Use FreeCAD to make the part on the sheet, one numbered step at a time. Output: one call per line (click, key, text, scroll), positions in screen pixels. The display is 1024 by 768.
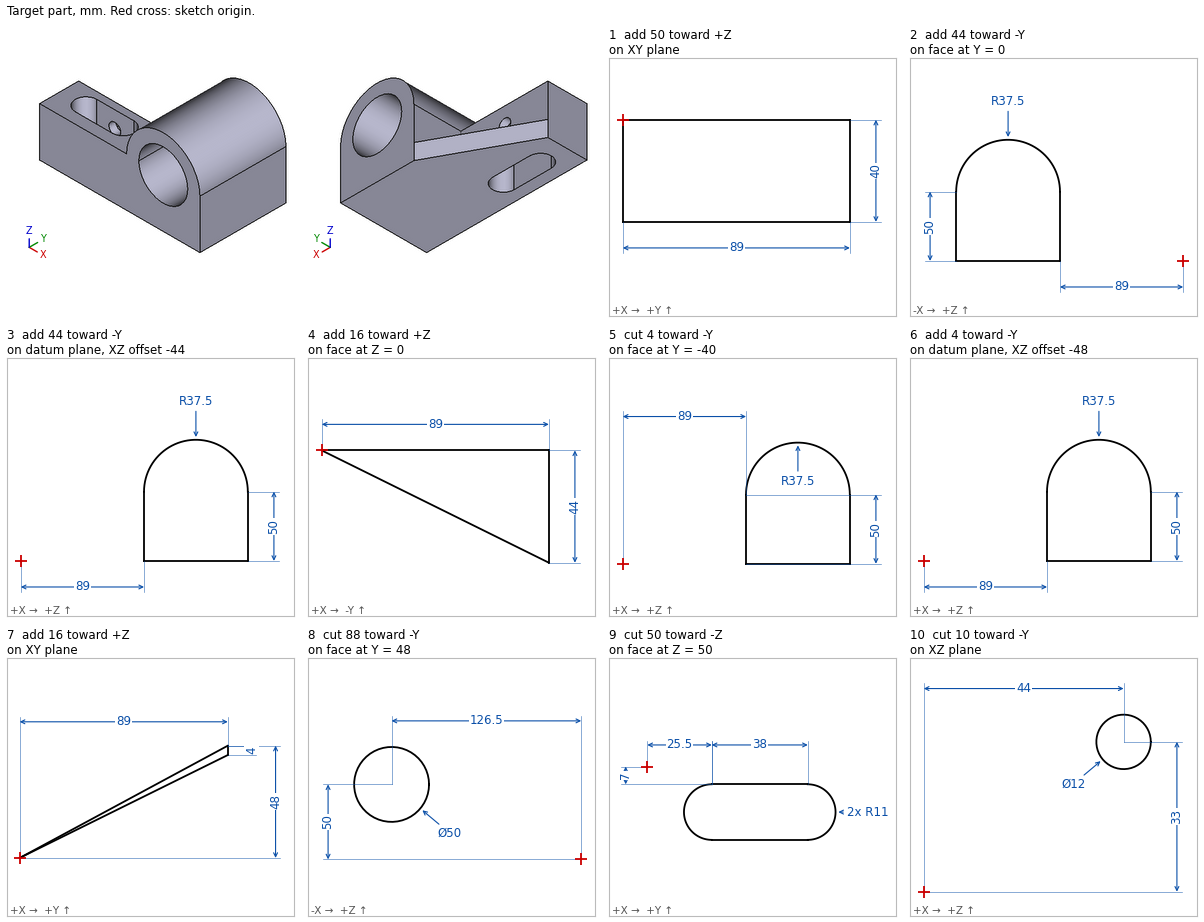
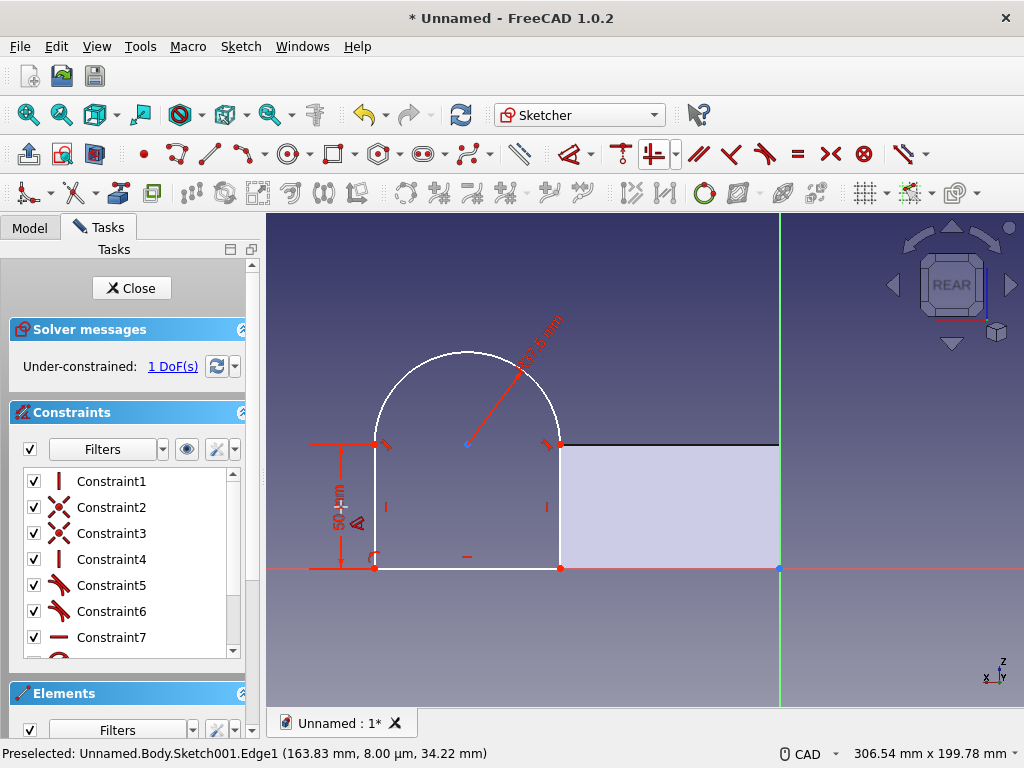
click(560, 569)
click(670, 603)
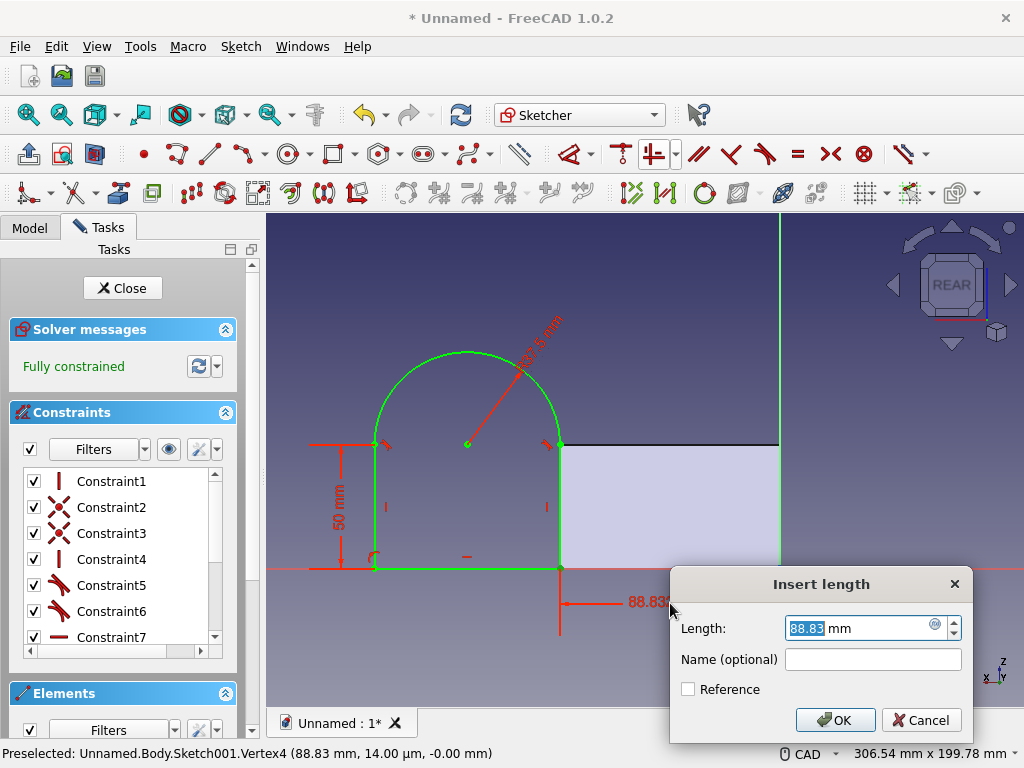
text(89)
key(Return)
key(Escape)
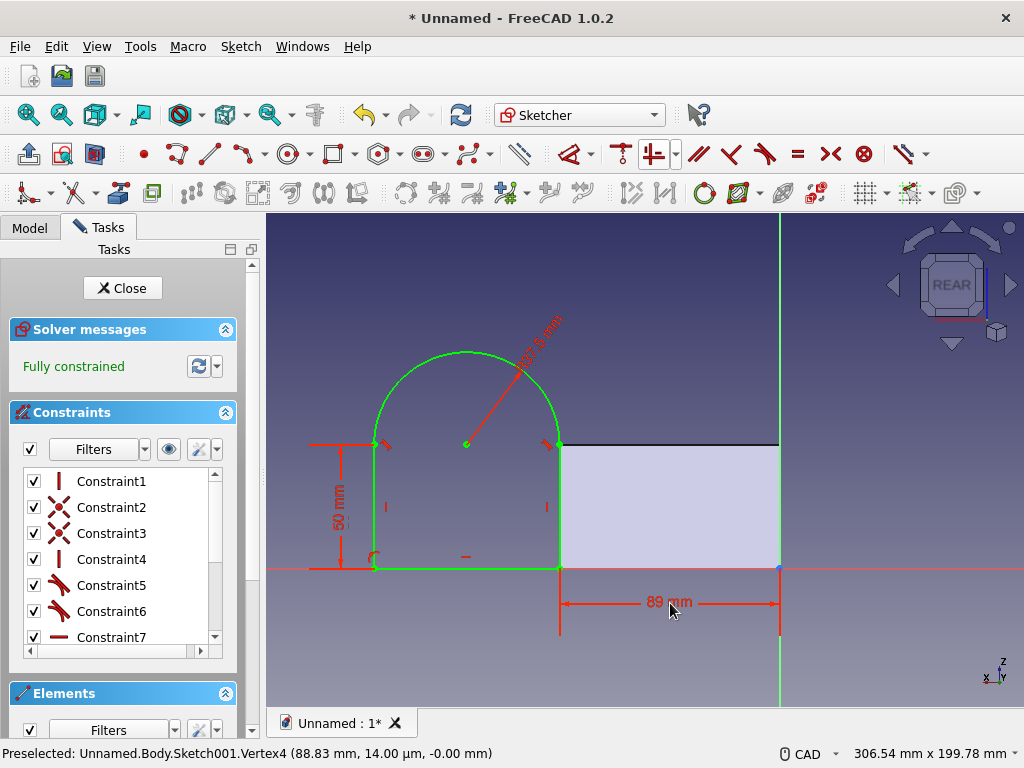
click(123, 288)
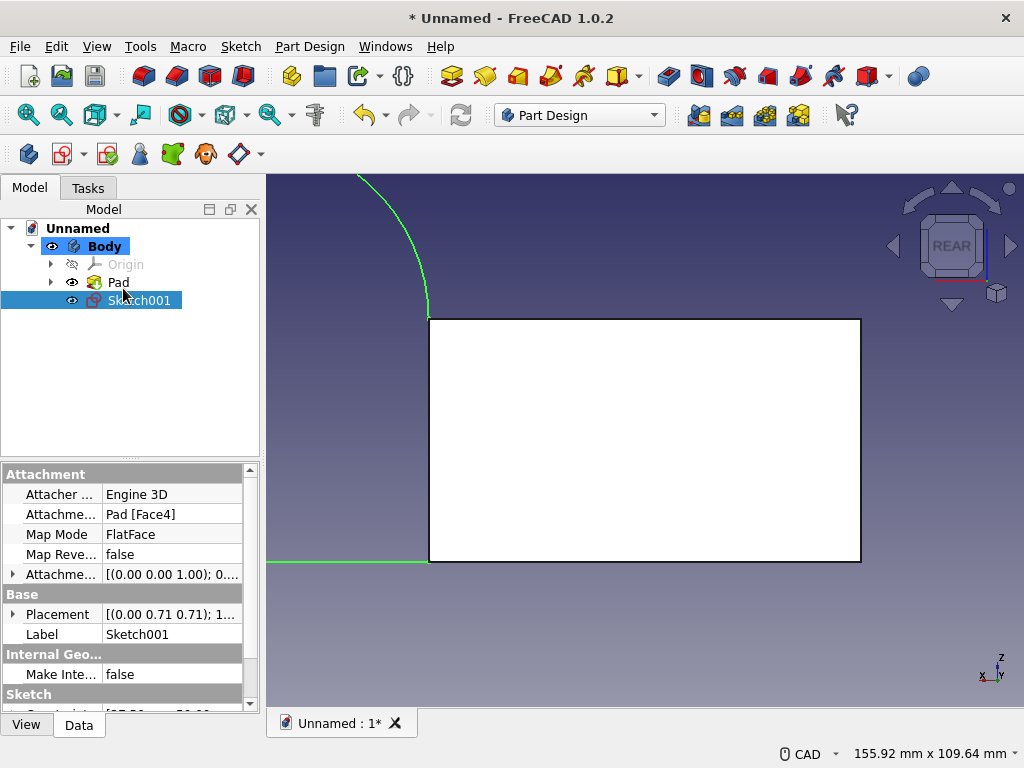
click(452, 76)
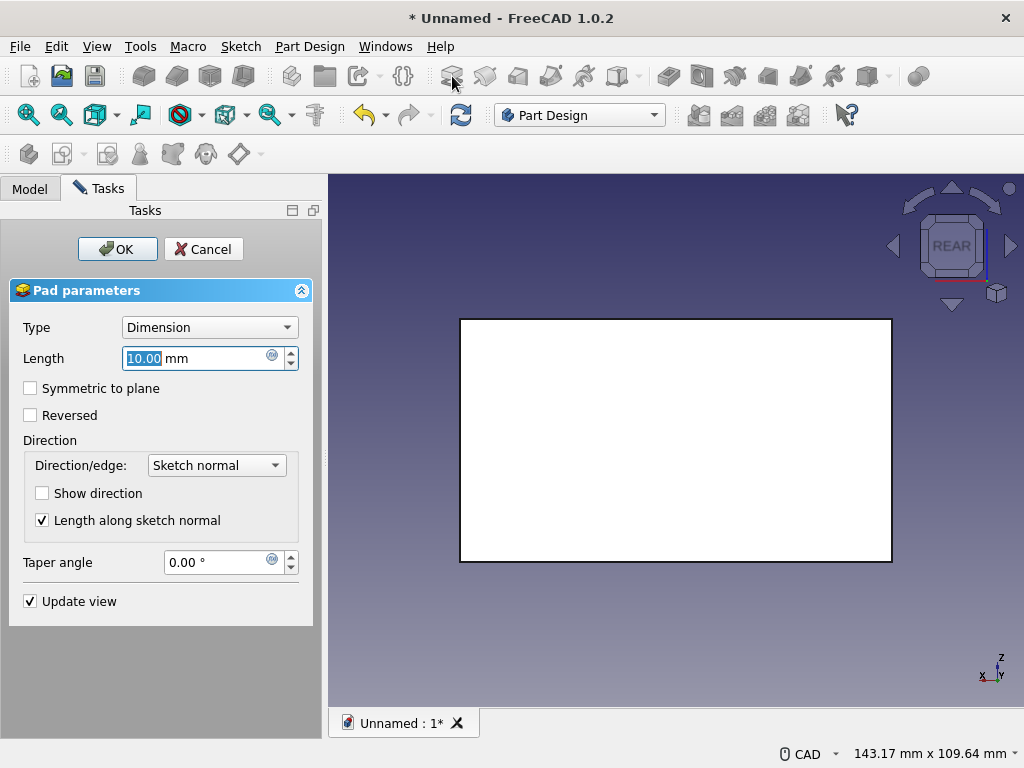
text(44)
key(Tab)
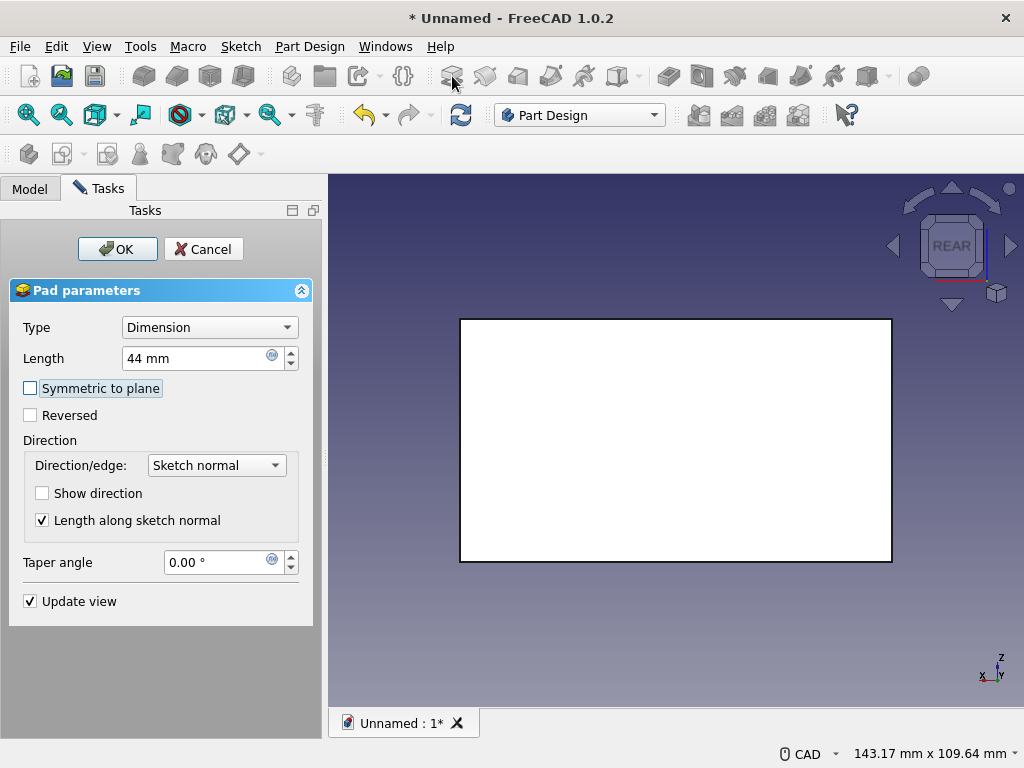
click(31, 415)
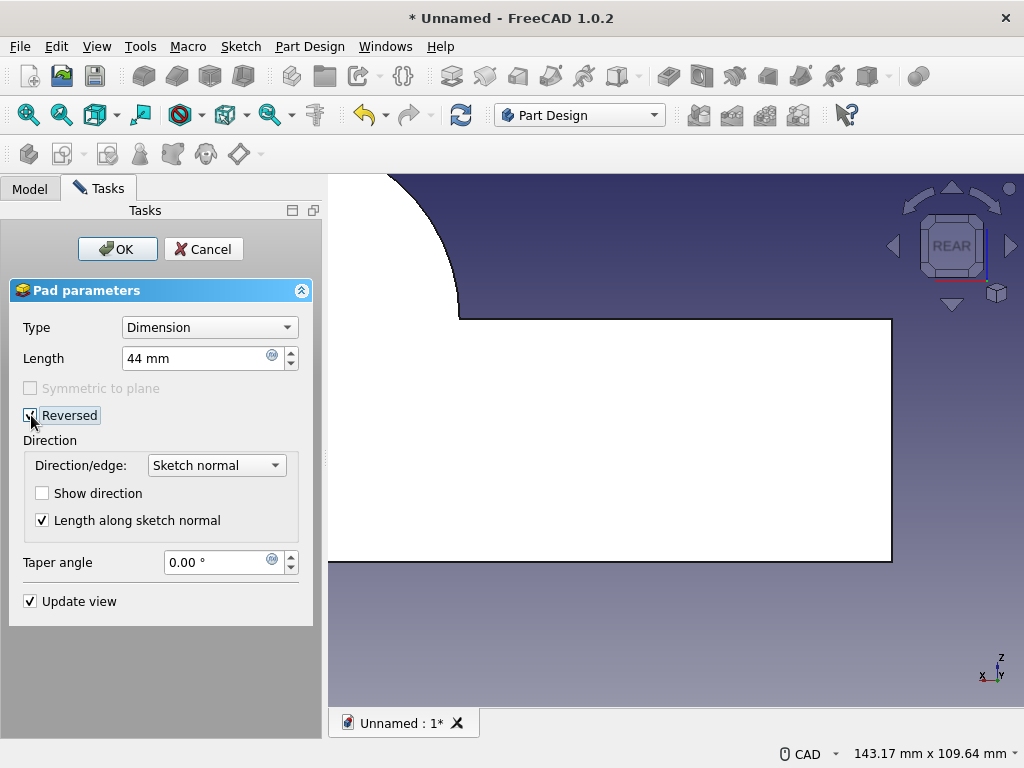
click(118, 249)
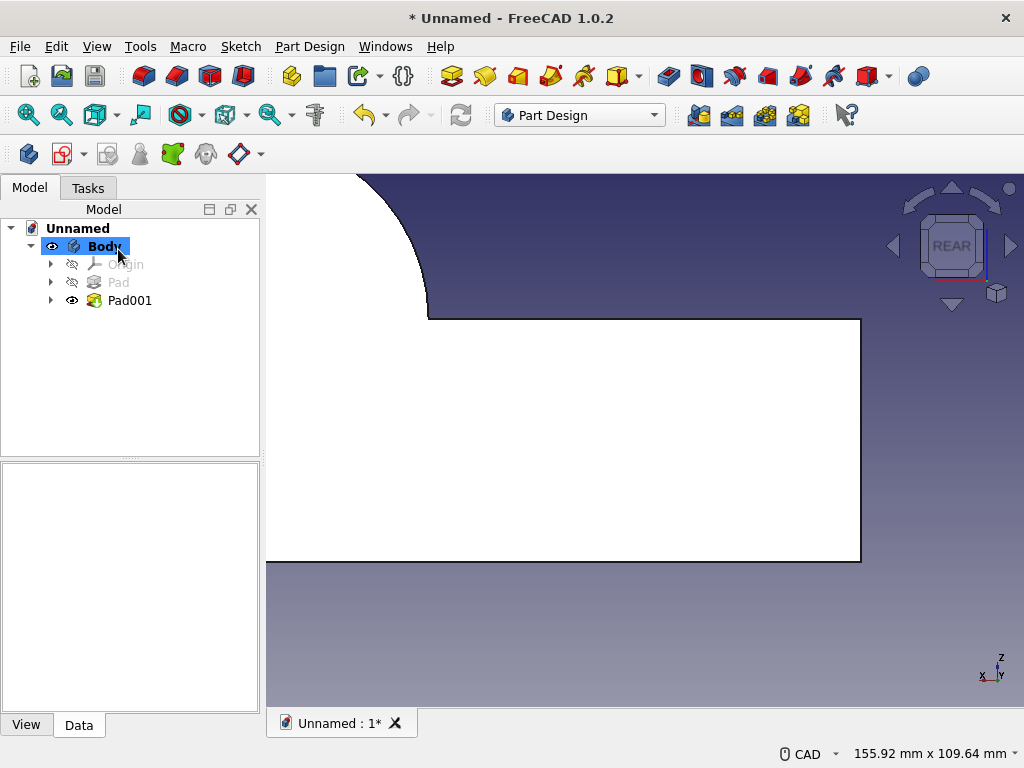
key(v)
key(f)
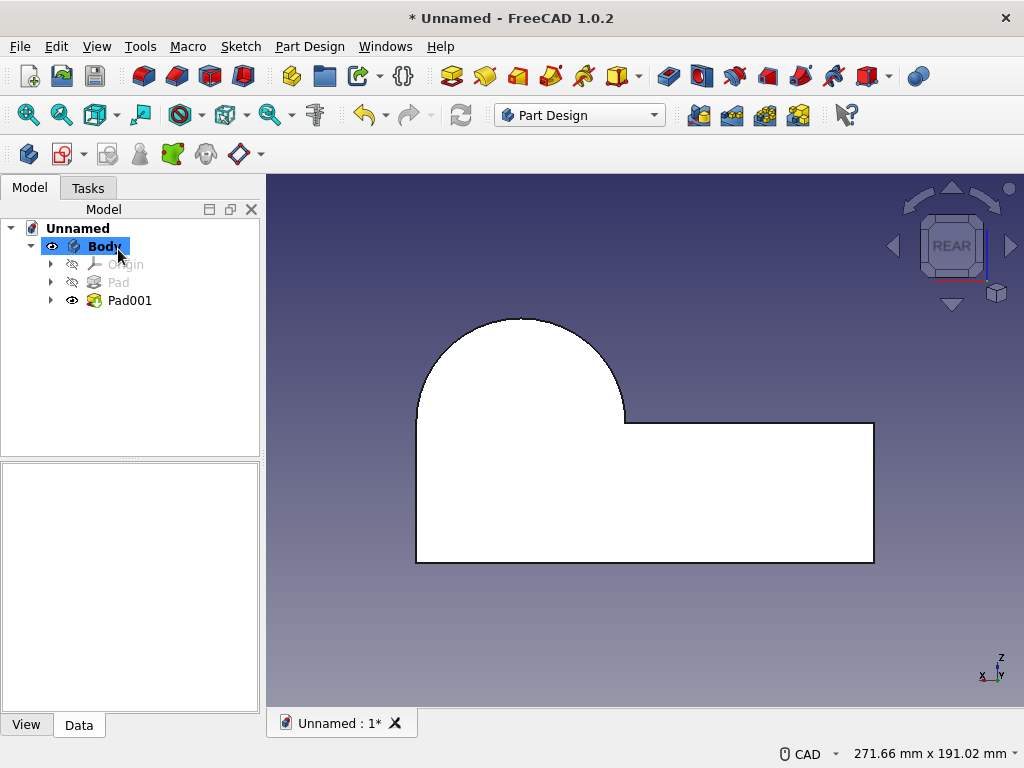
click(51, 264)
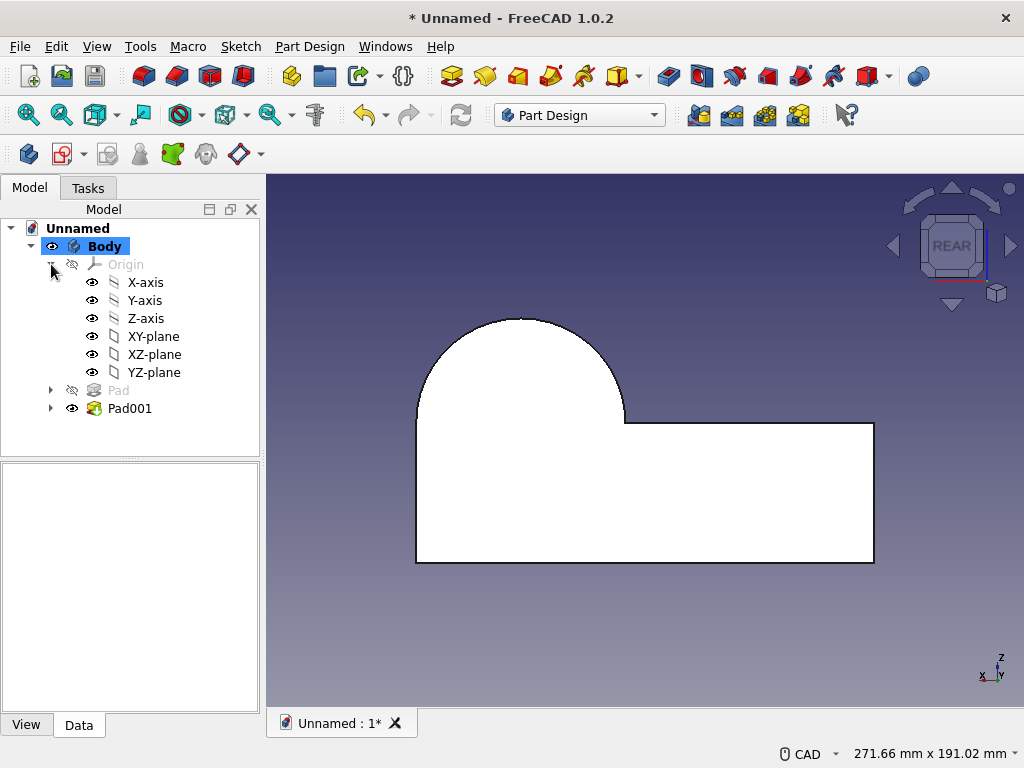
click(137, 354)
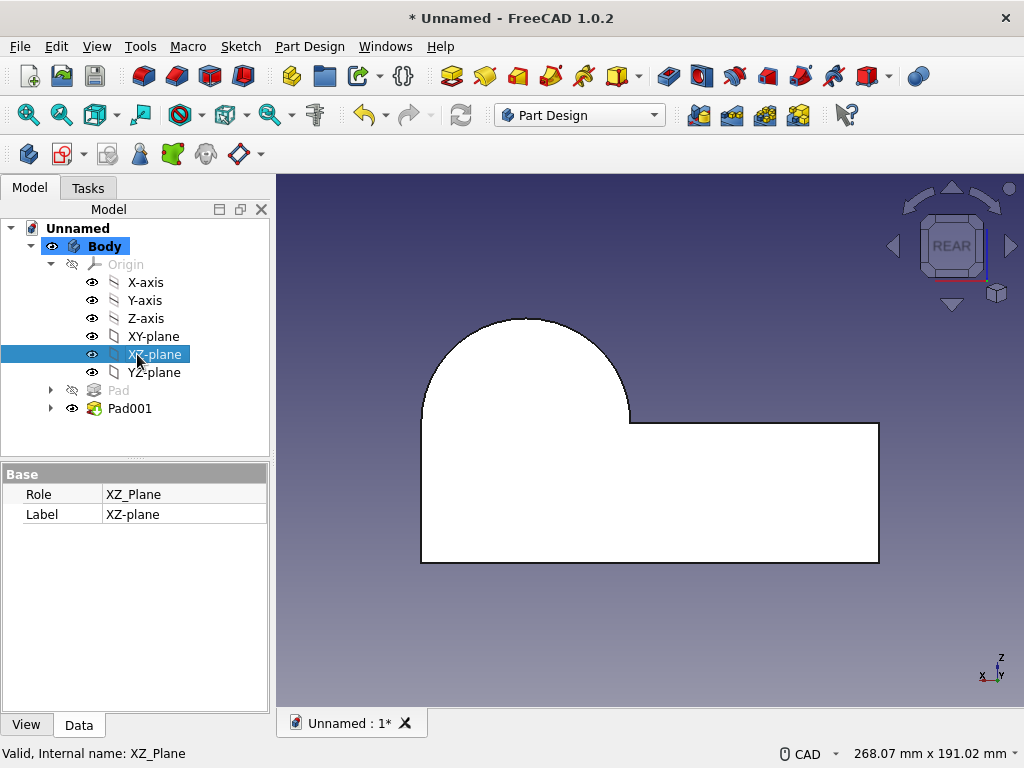
click(238, 154)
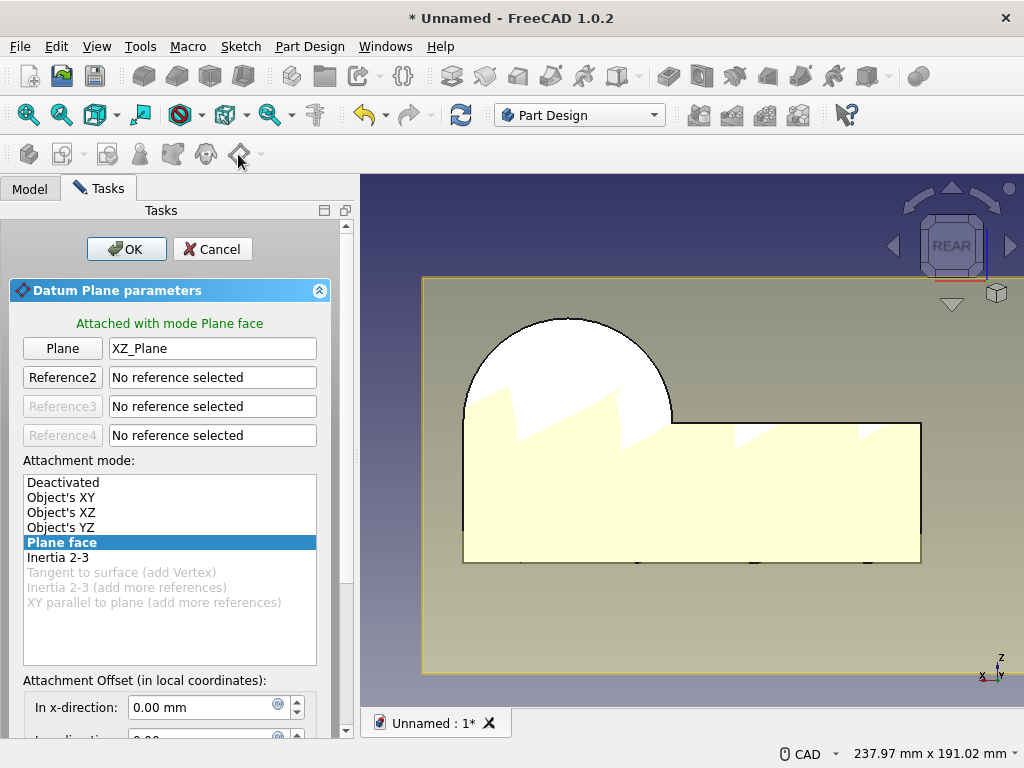
scroll(346, 479, down, 2)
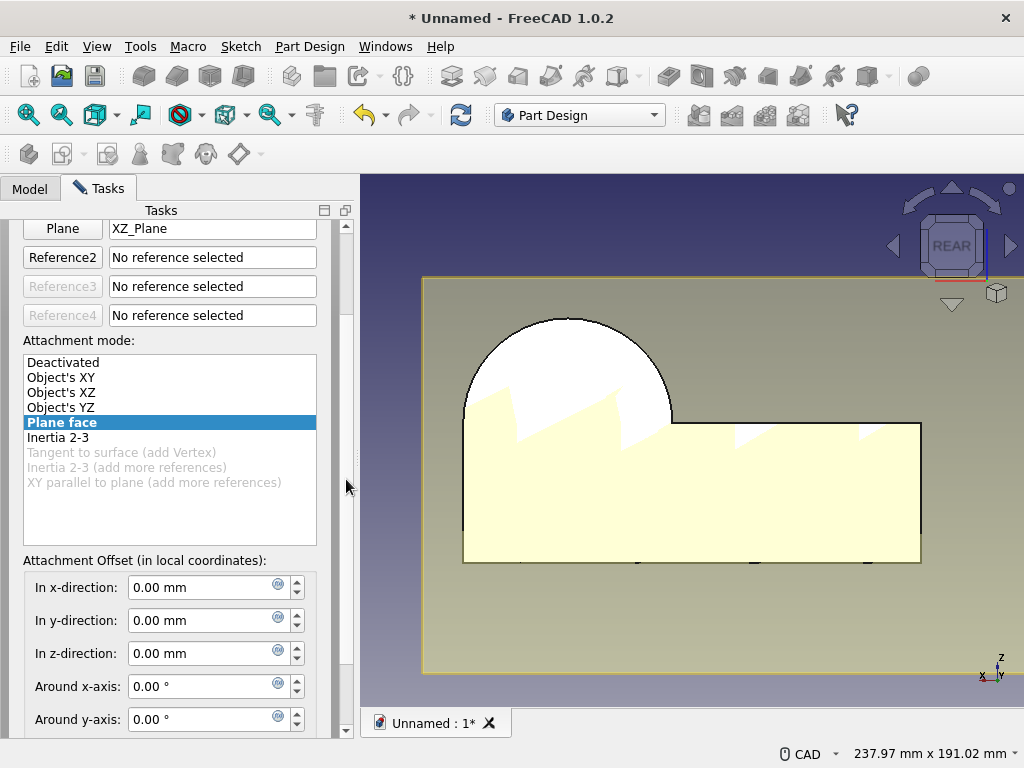
triple_click(210, 654)